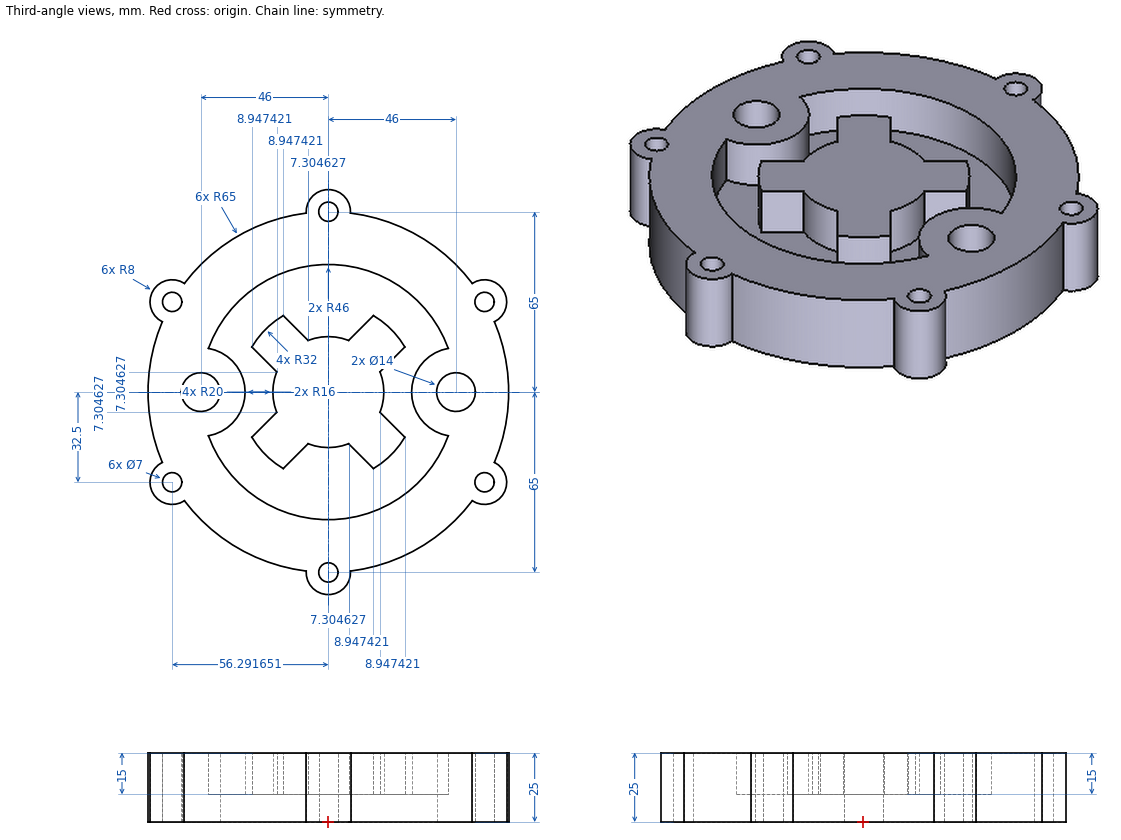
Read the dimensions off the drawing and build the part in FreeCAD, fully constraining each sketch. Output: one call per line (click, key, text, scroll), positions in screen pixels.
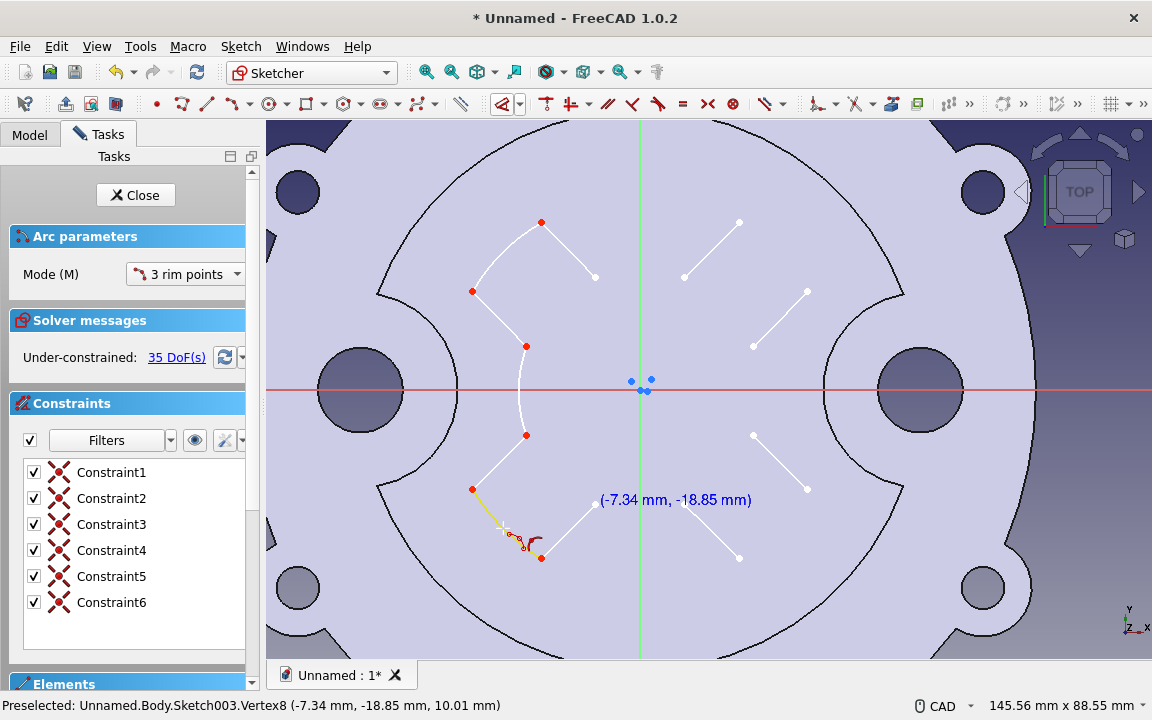
click(685, 505)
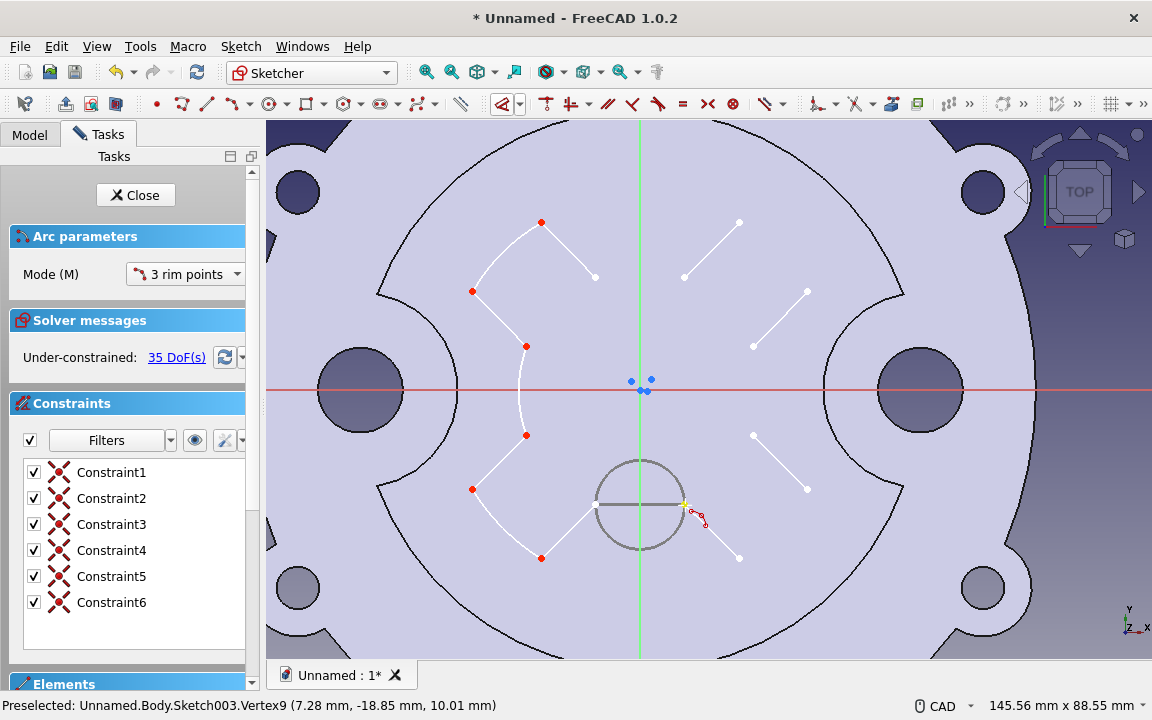
scroll(631, 512, up, 4)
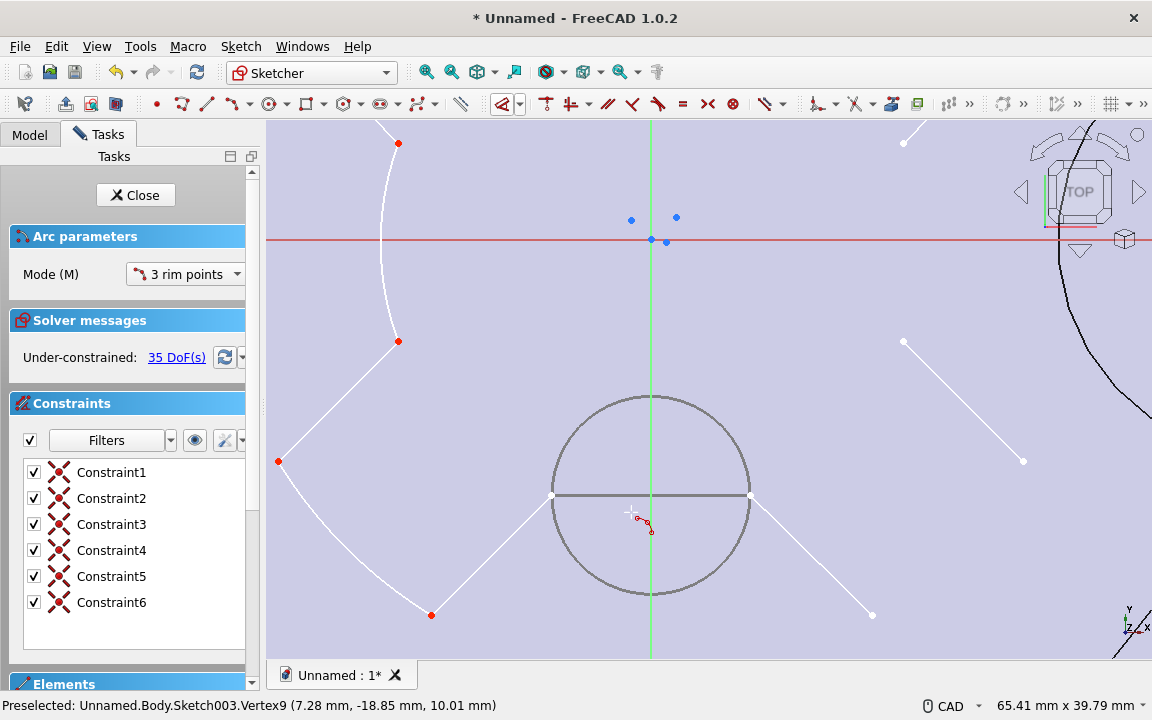
click(631, 510)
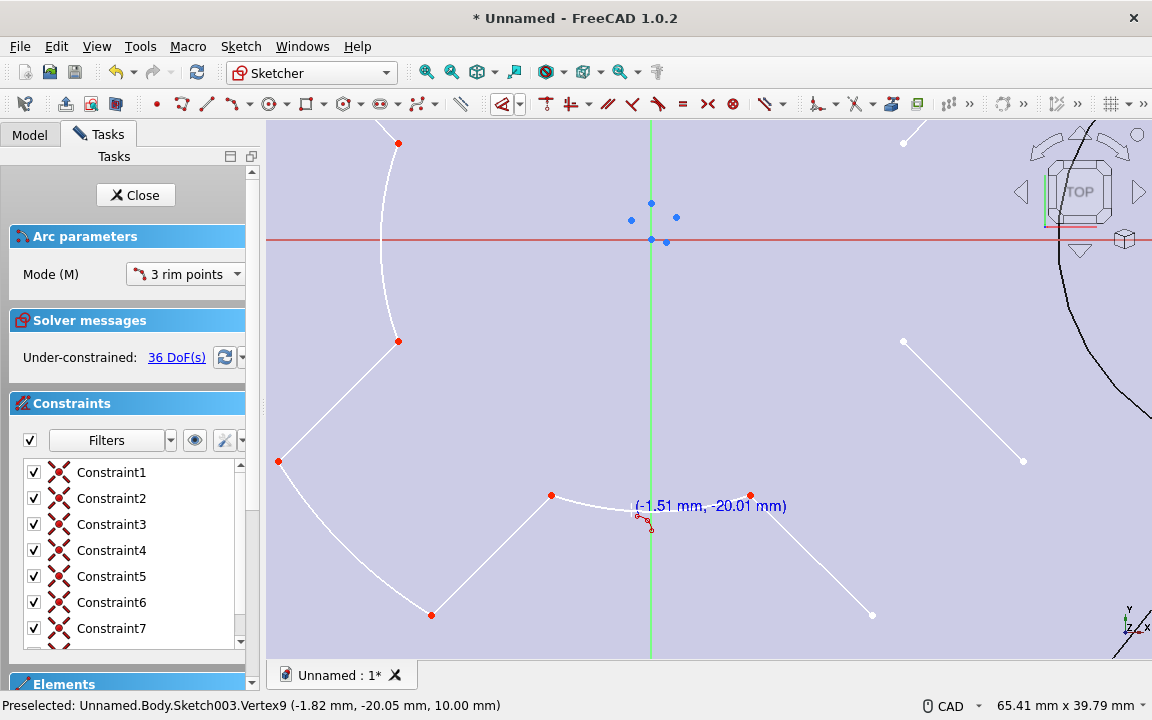
click(872, 615)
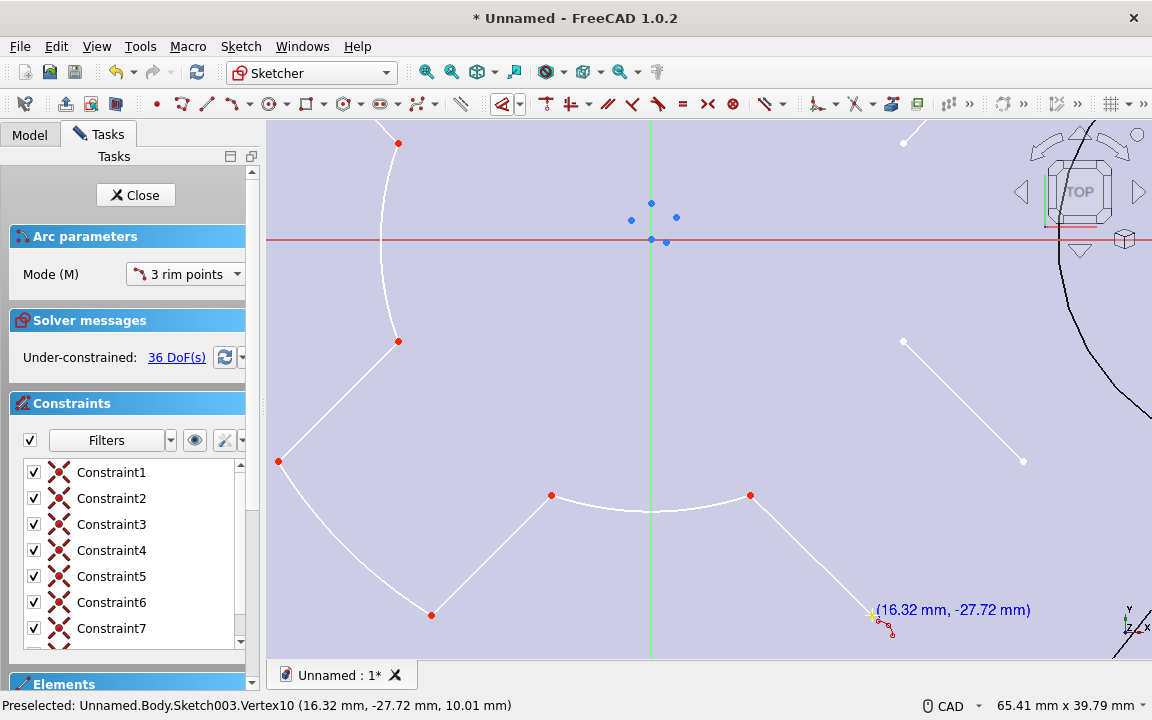
scroll(632, 512, down, 4)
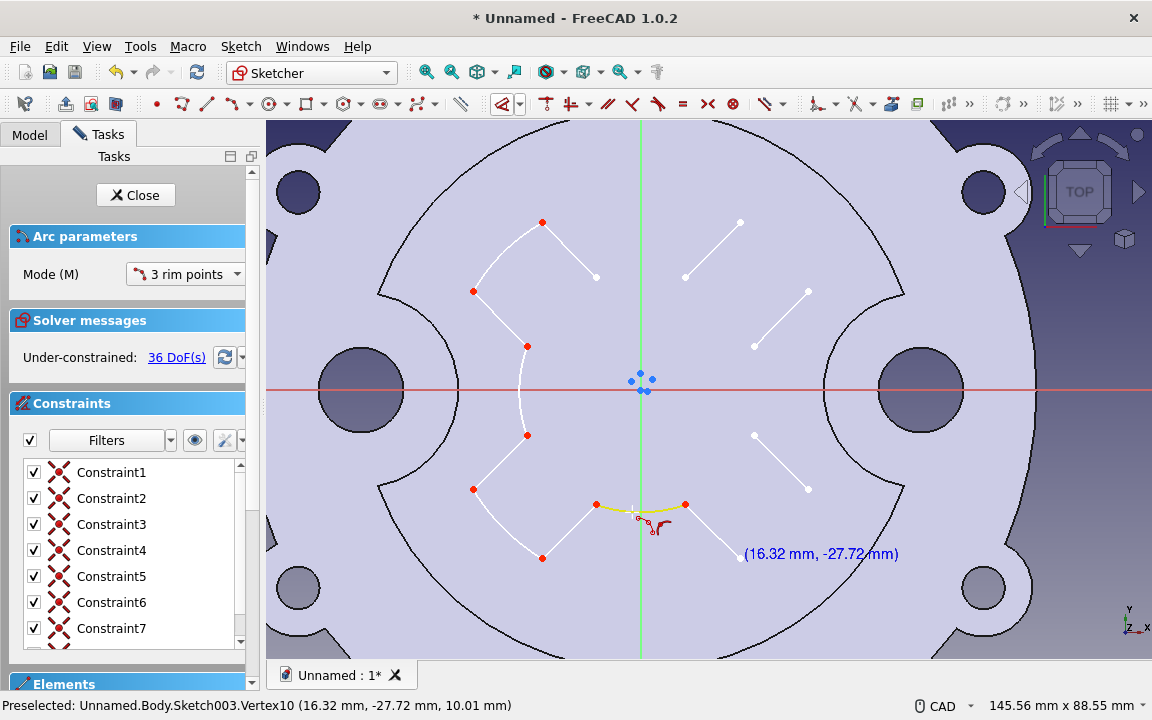
click(808, 490)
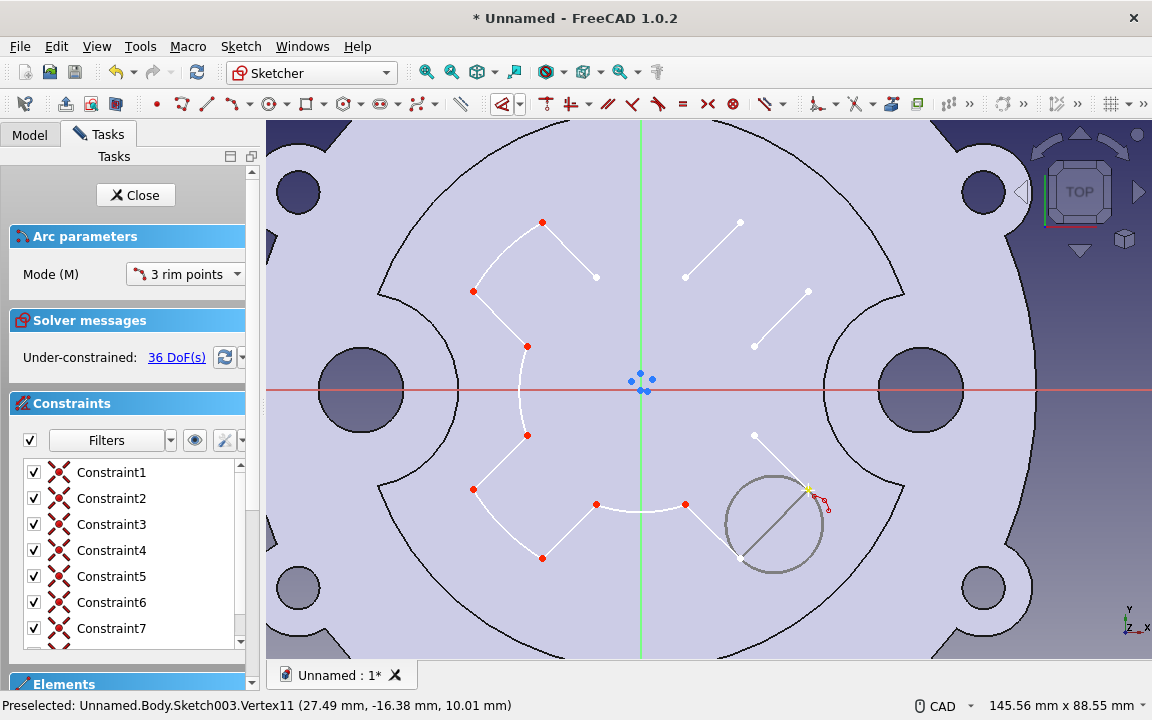
scroll(779, 528, up, 5)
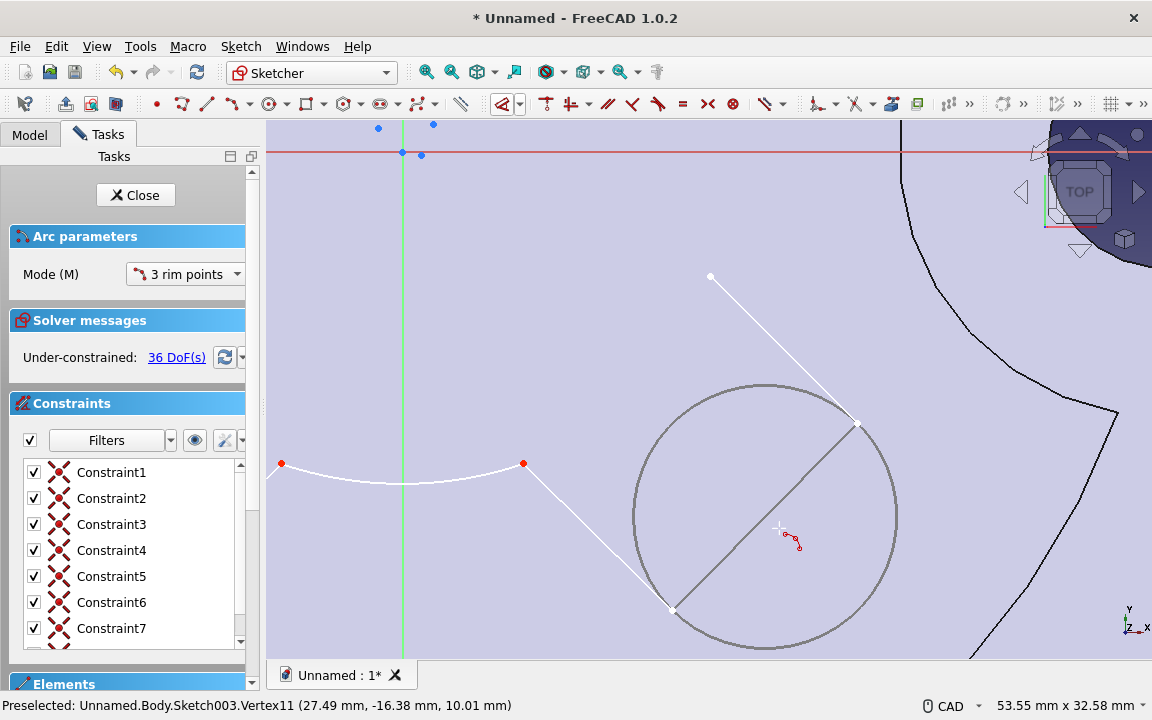
click(777, 526)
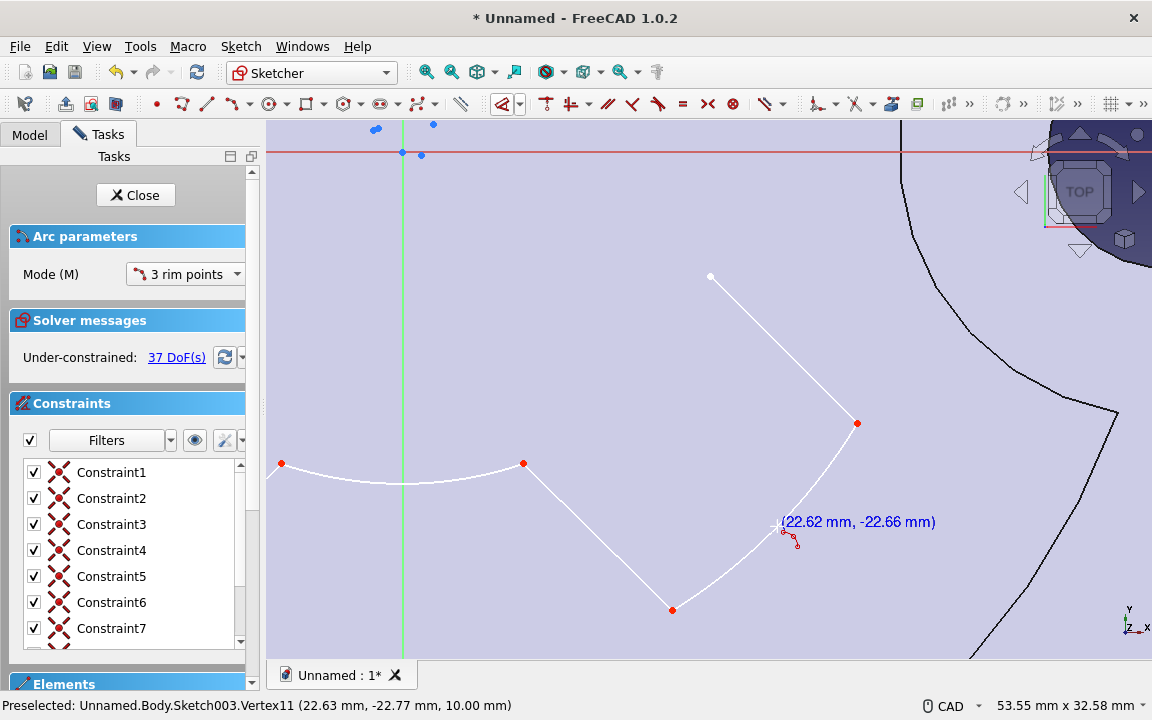
click(711, 276)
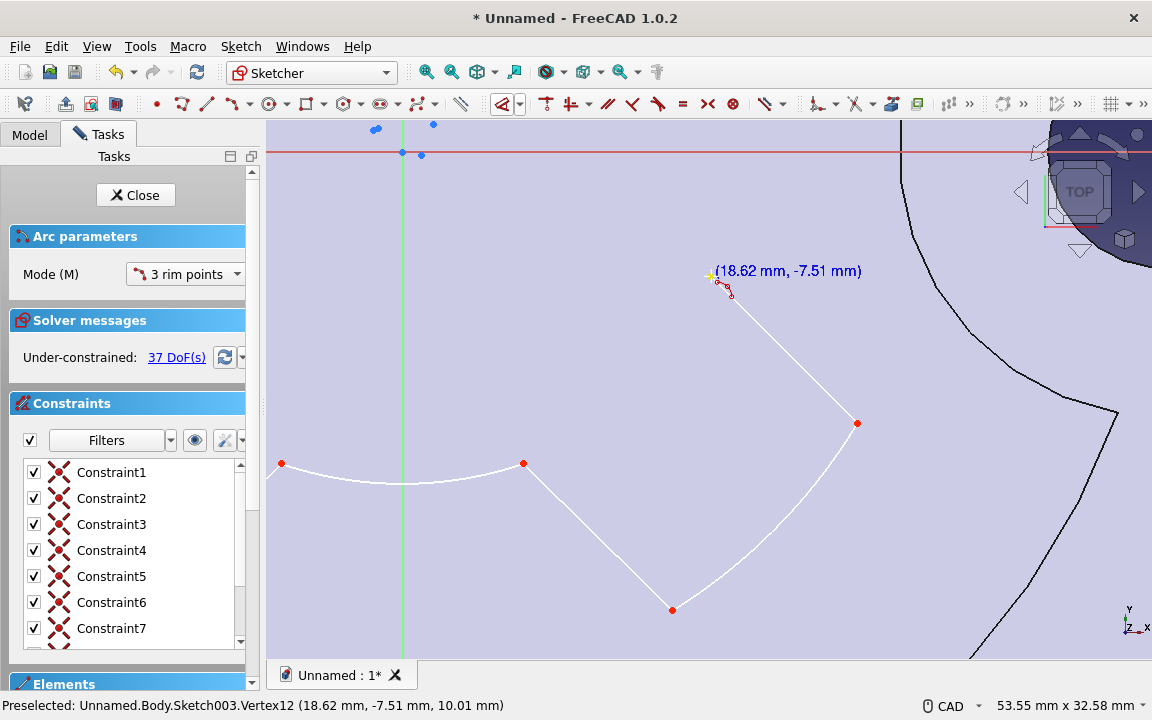
scroll(779, 528, down, 5)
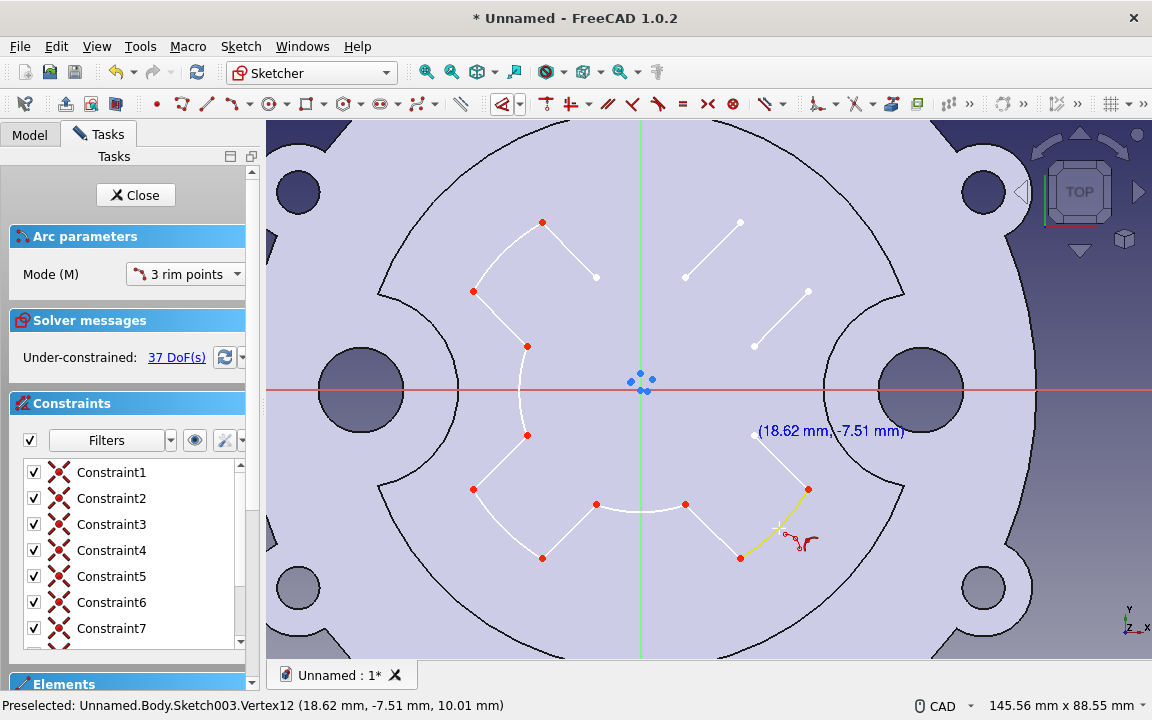
click(754, 347)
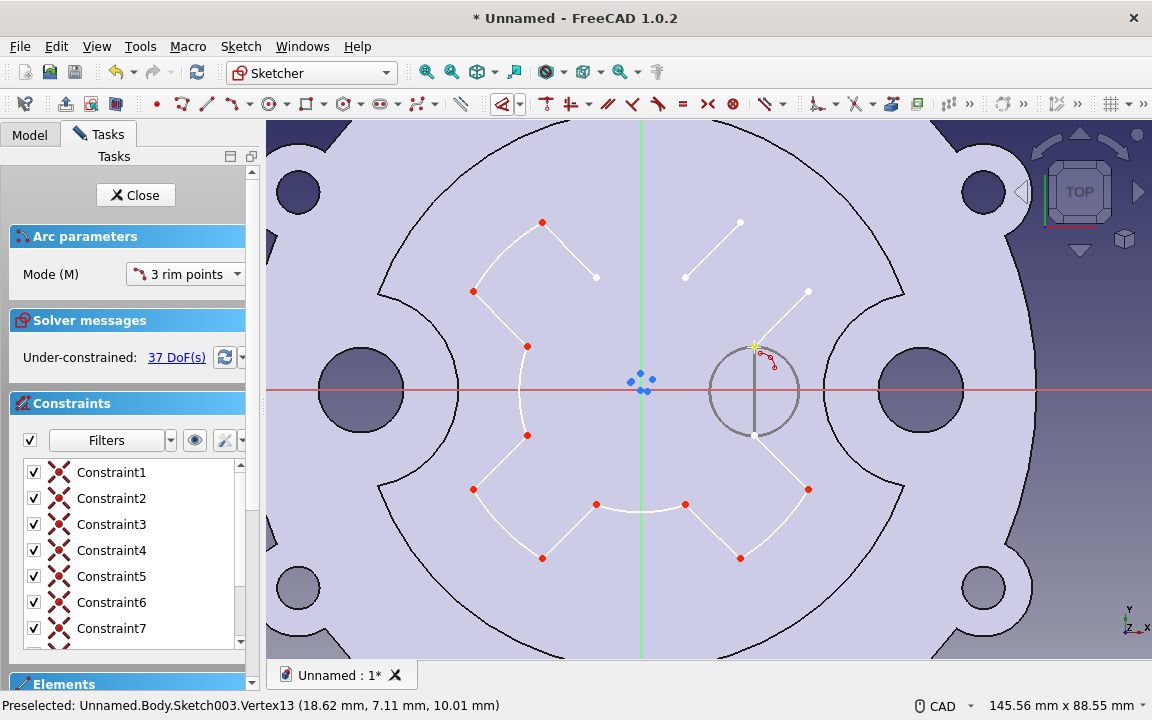
scroll(762, 399, up, 4)